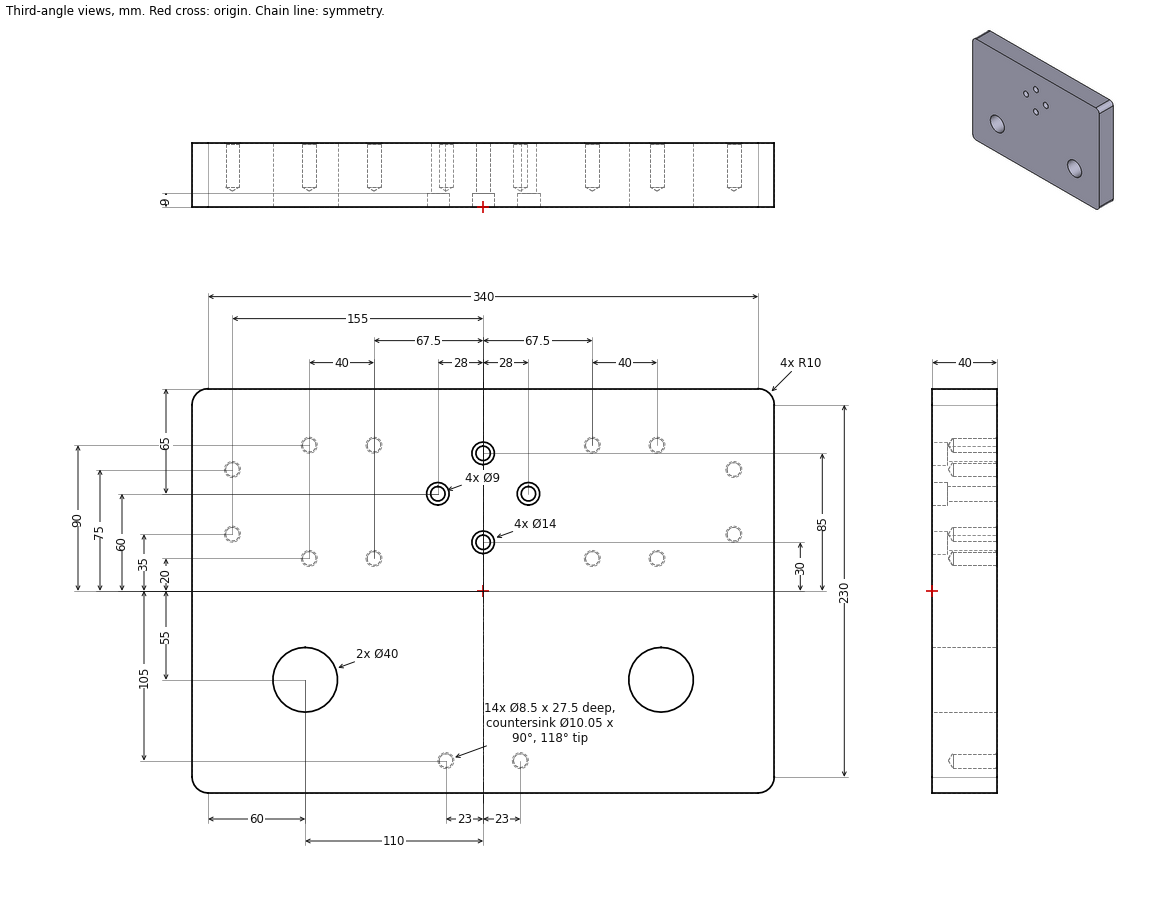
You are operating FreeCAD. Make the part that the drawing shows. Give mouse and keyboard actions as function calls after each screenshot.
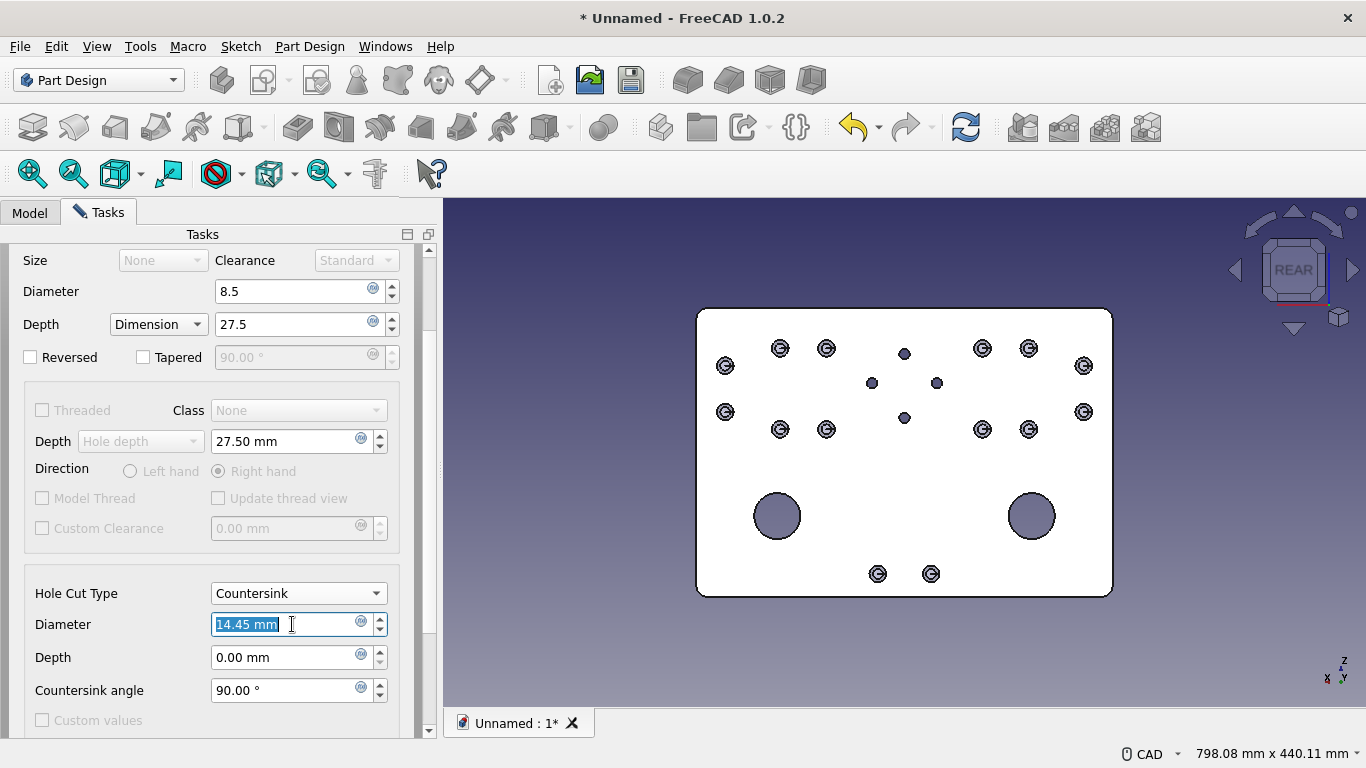
text(10.05)
key(Tab)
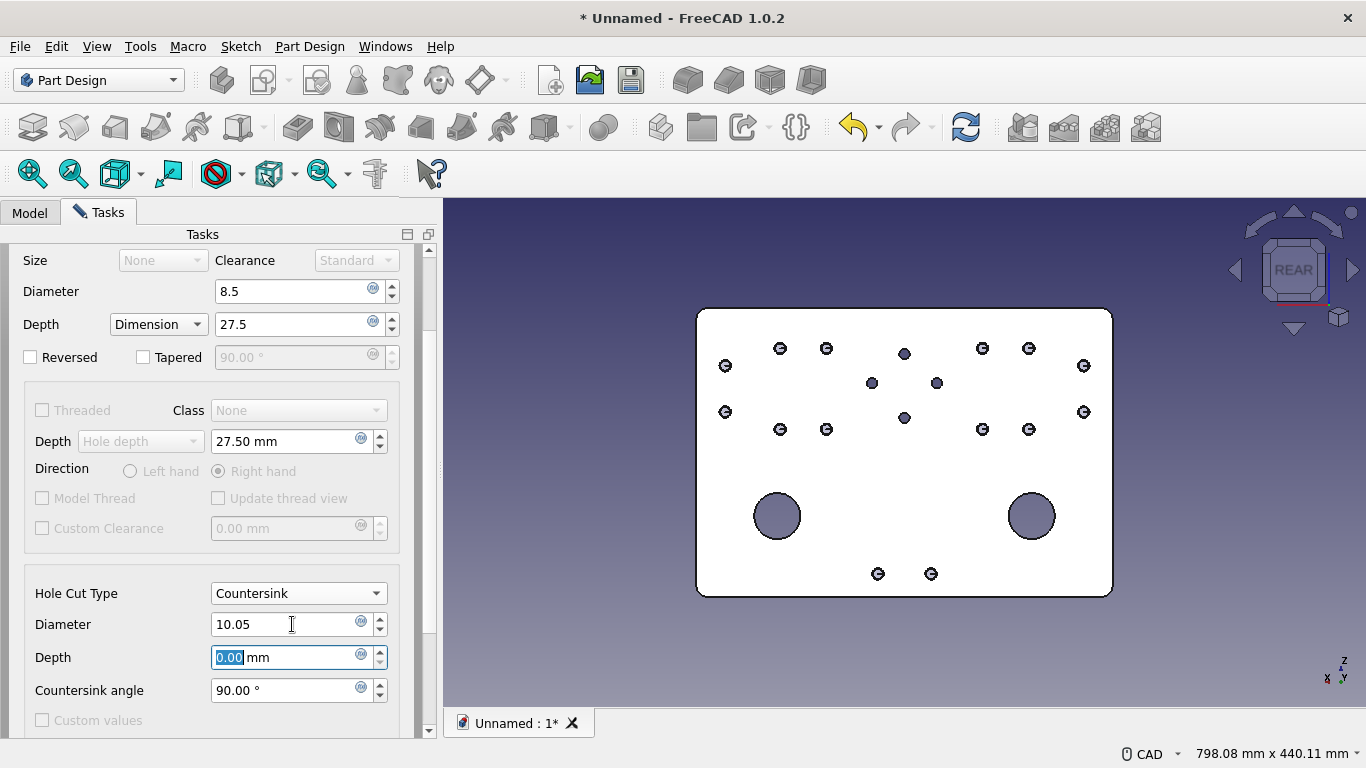
scroll(429, 491, up, 3)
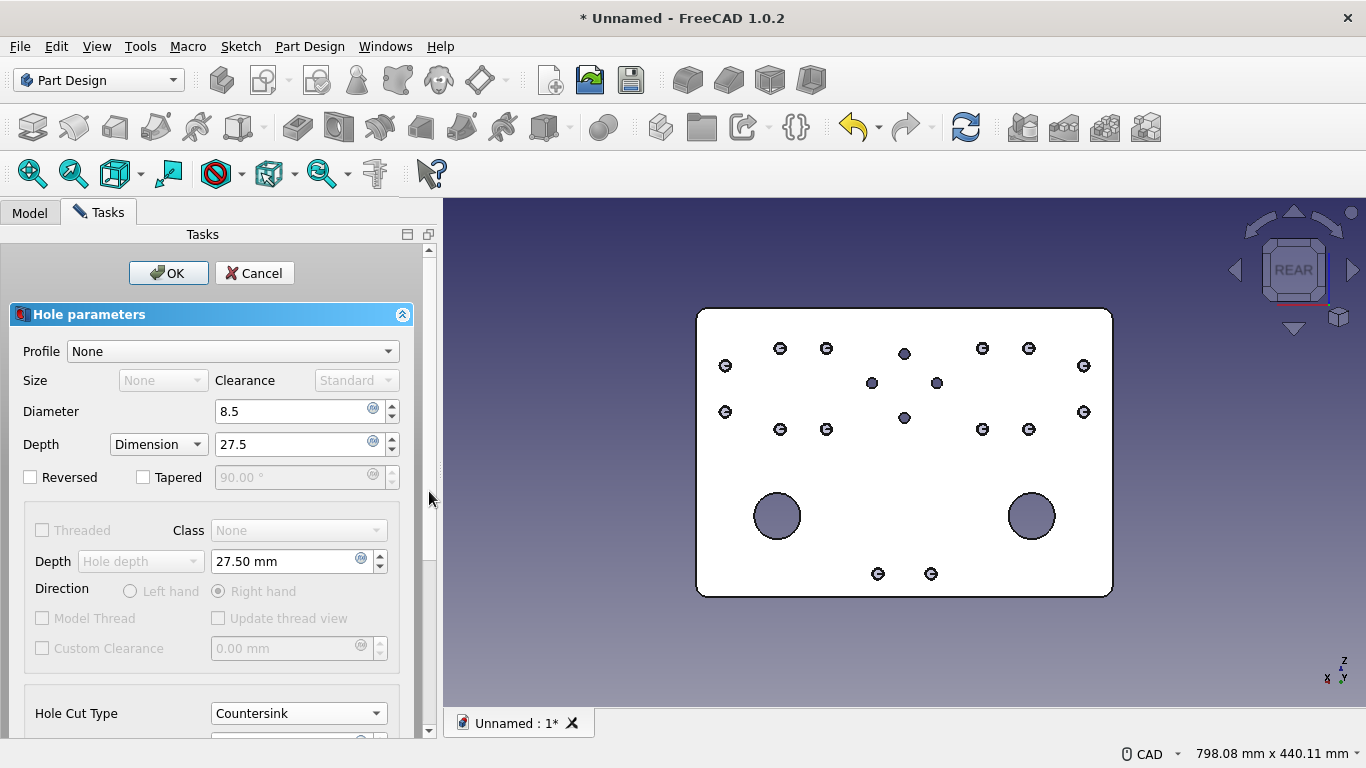
click(169, 273)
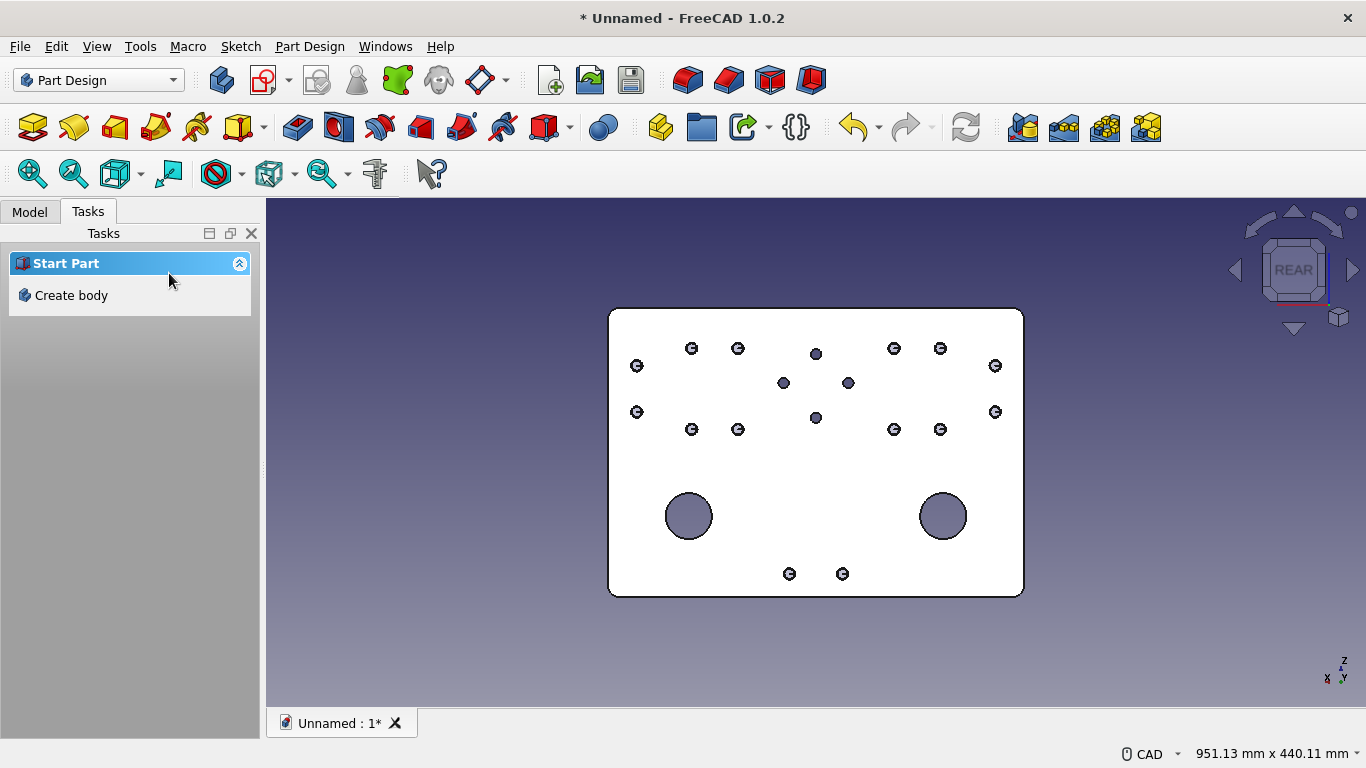
key(0)